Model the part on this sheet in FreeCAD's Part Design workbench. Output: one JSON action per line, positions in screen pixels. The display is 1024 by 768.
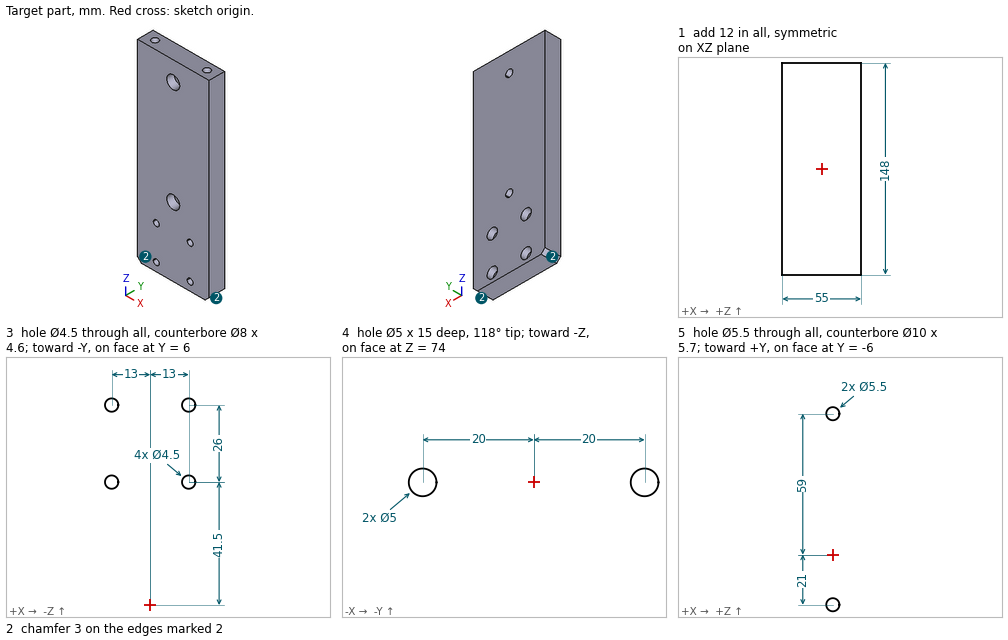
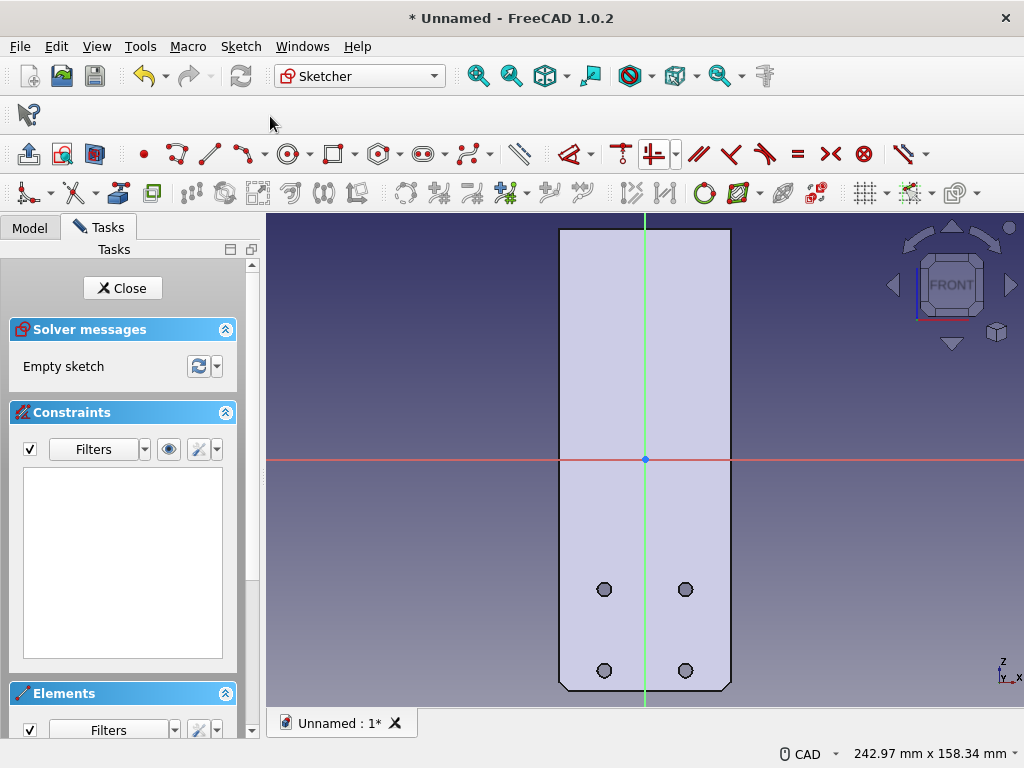
{"action": "key", "text": "g c"}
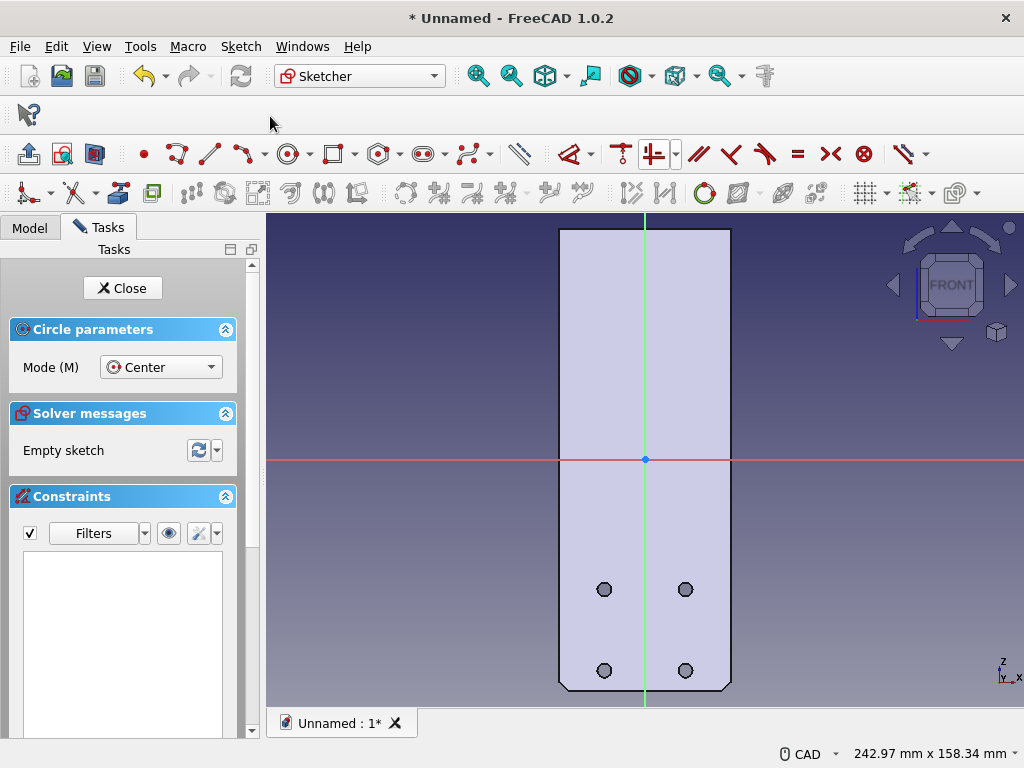
{"action": "scroll", "coordinate": [645, 276], "scroll_direction": "up", "scroll_amount": 5}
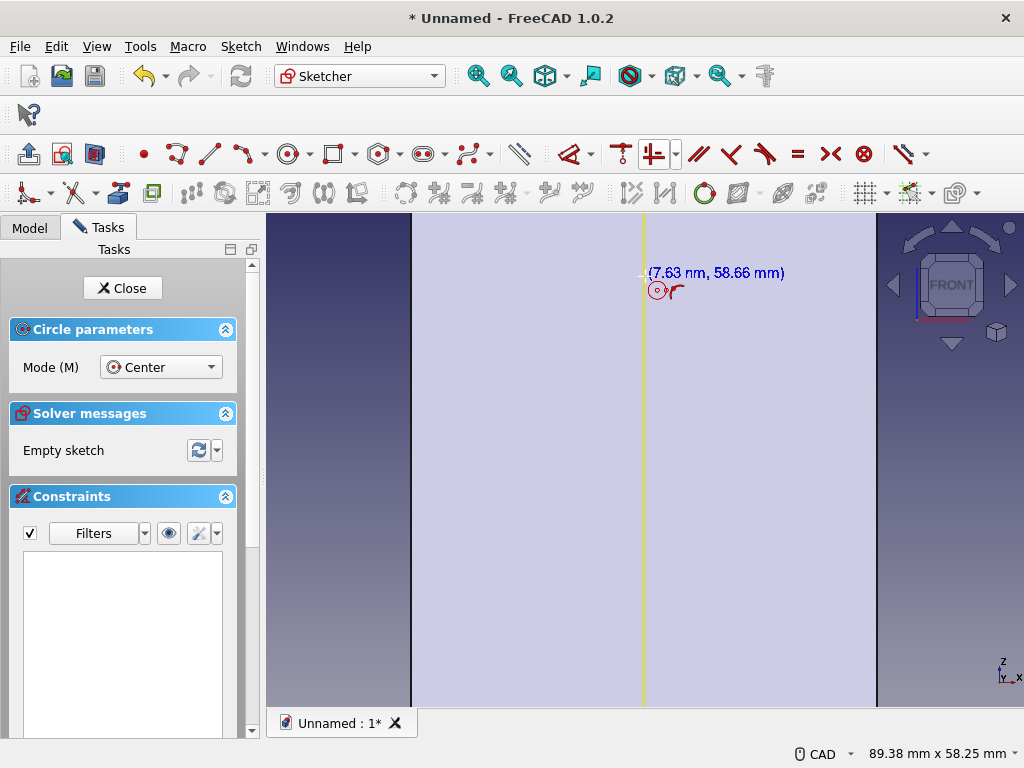
{"action": "left_click", "coordinate": [644, 276]}
{"action": "mouse_move", "coordinate": [661, 259]}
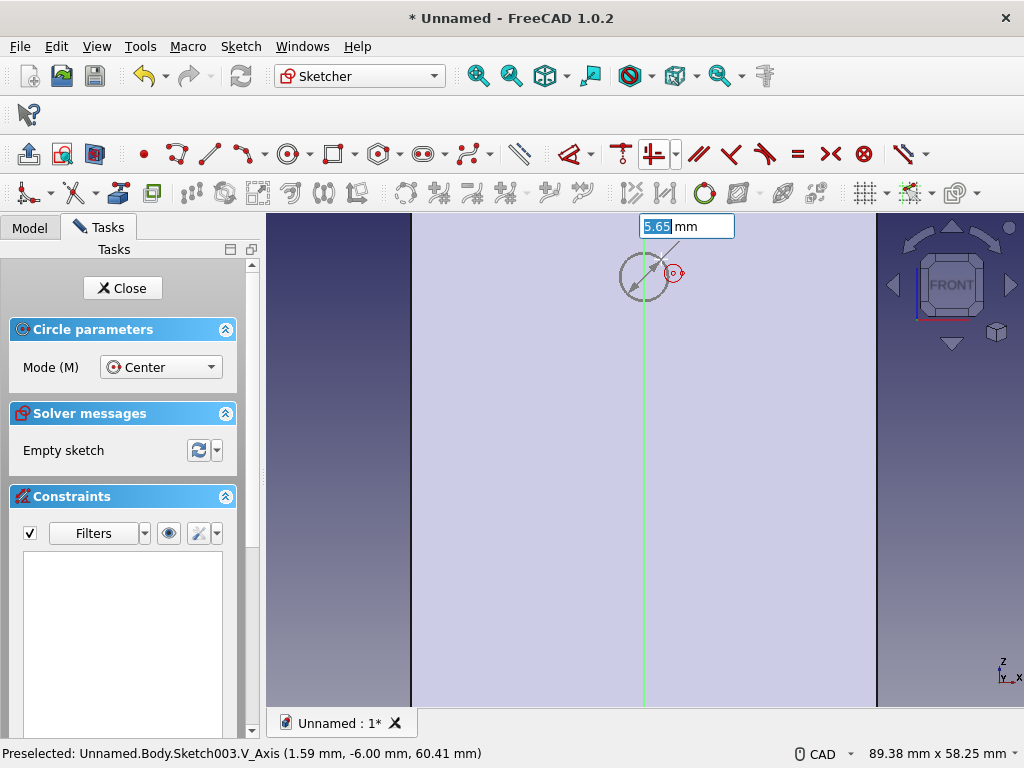
{"action": "type", "text": "5.5"}
{"action": "key", "text": "Return"}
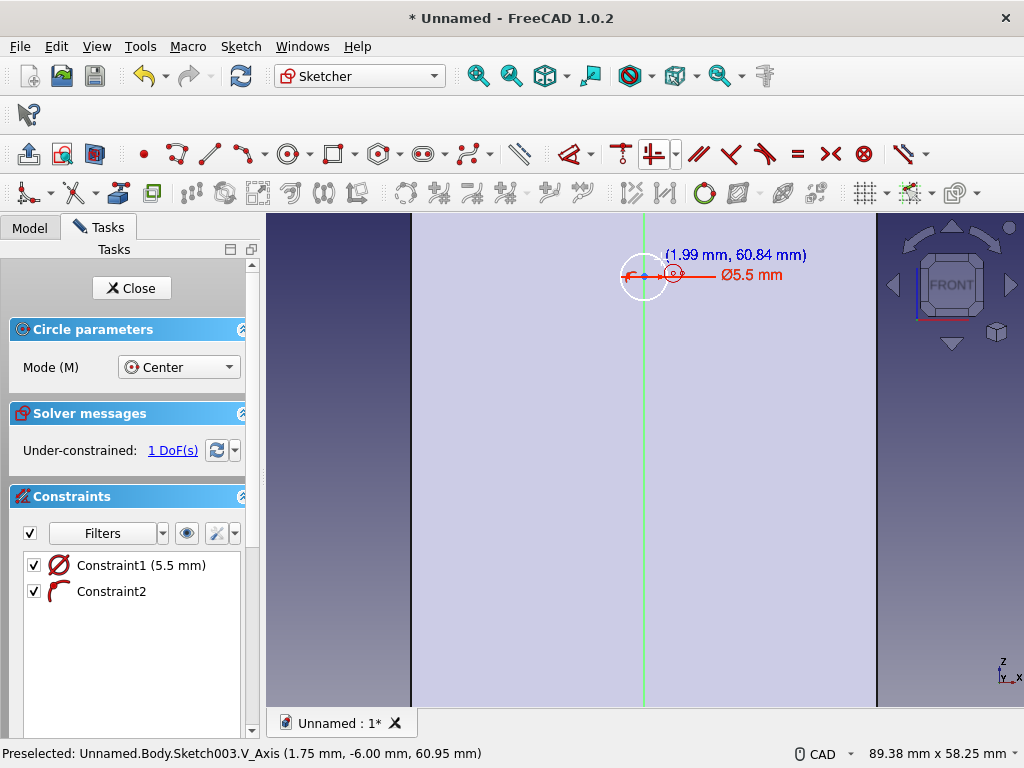
{"action": "scroll", "coordinate": [521, 334], "scroll_direction": "down", "scroll_amount": 4}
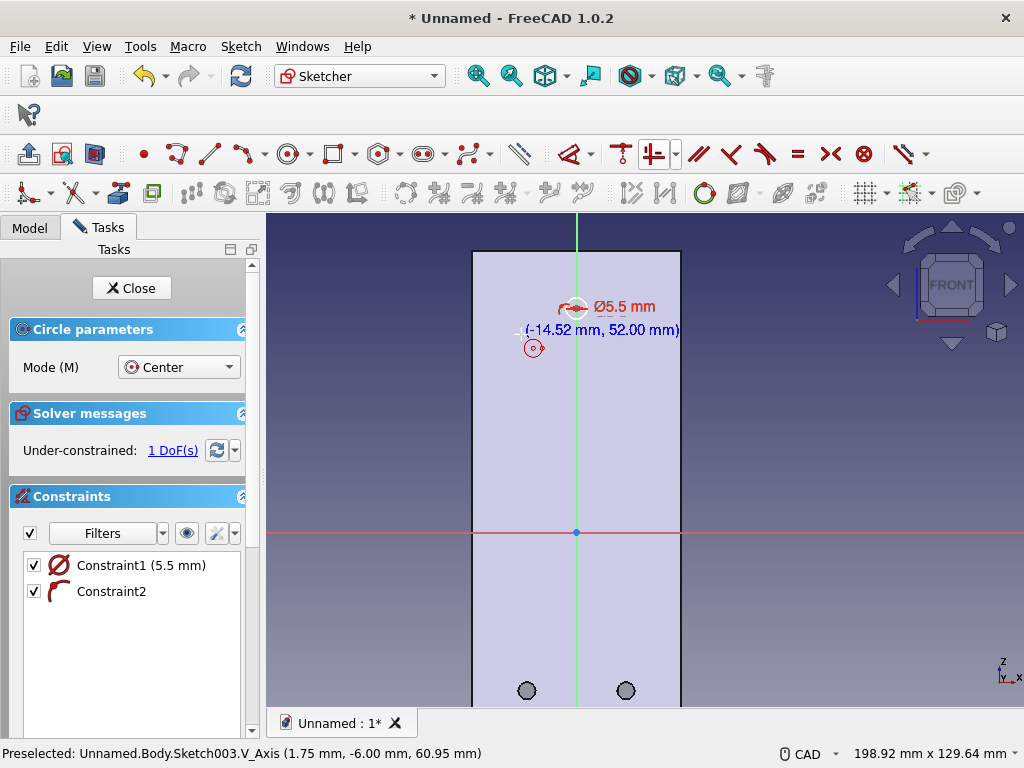
{"action": "scroll", "coordinate": [577, 613], "scroll_direction": "up", "scroll_amount": 4}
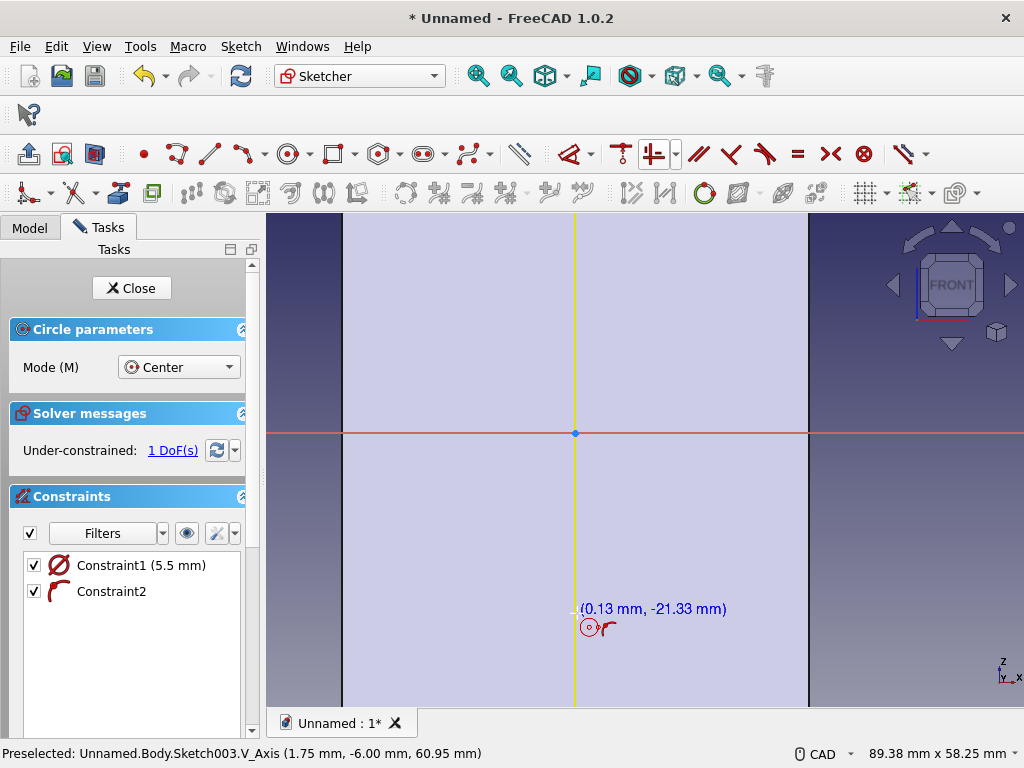
{"action": "left_click", "coordinate": [575, 611]}
{"action": "mouse_move", "coordinate": [592, 595]}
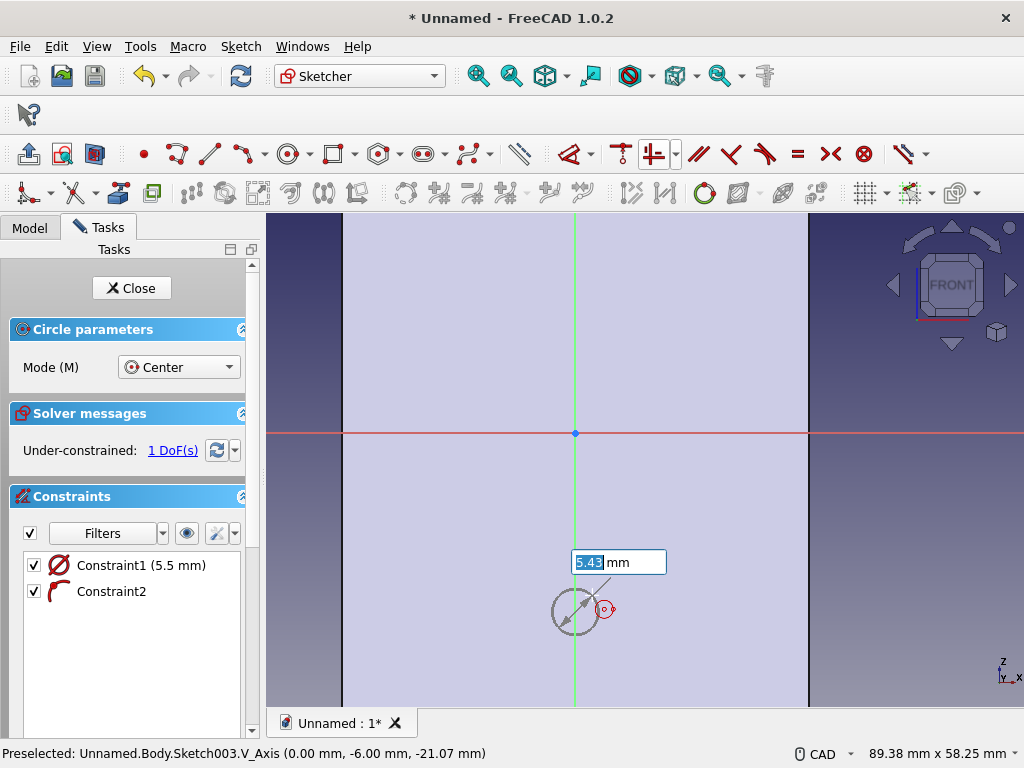
{"action": "type", "text": "5.5"}
{"action": "key", "text": "Return"}
{"action": "key", "text": "Escape"}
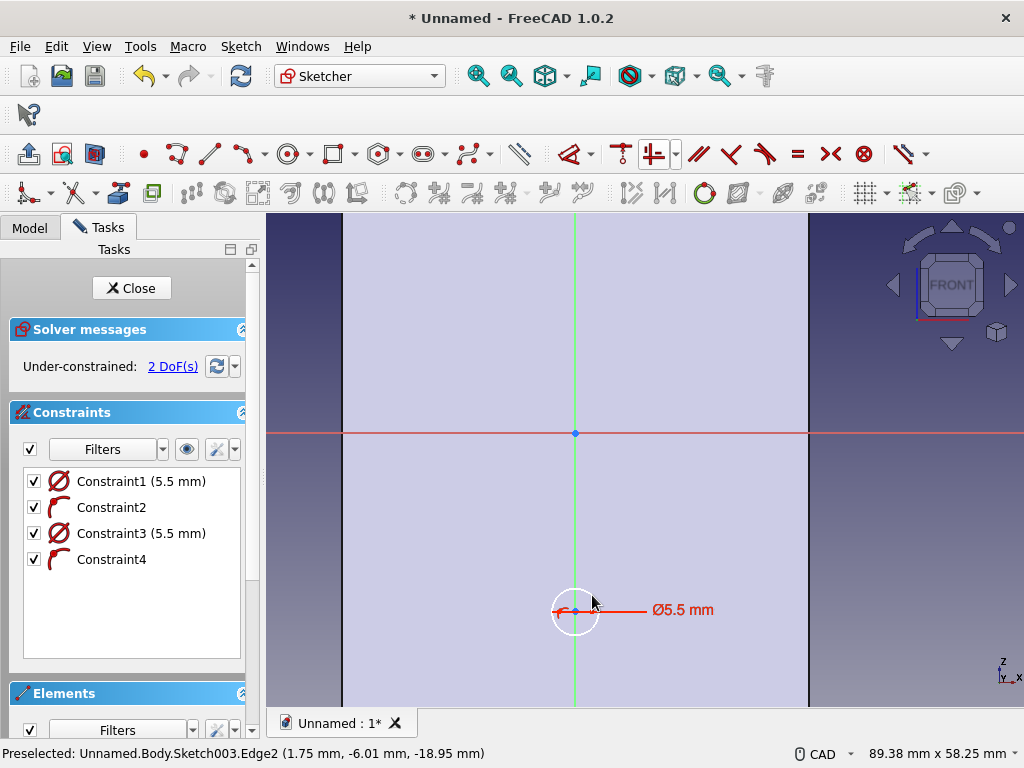
{"action": "key", "text": "d"}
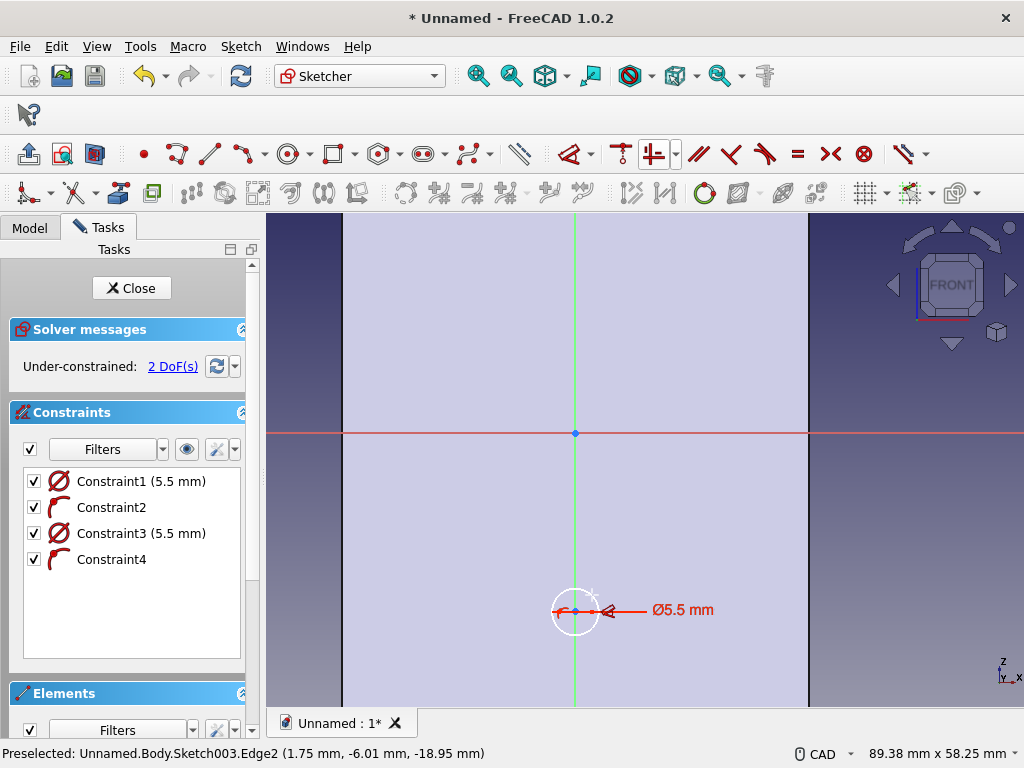
{"action": "scroll", "coordinate": [577, 613], "scroll_direction": "down", "scroll_amount": 4}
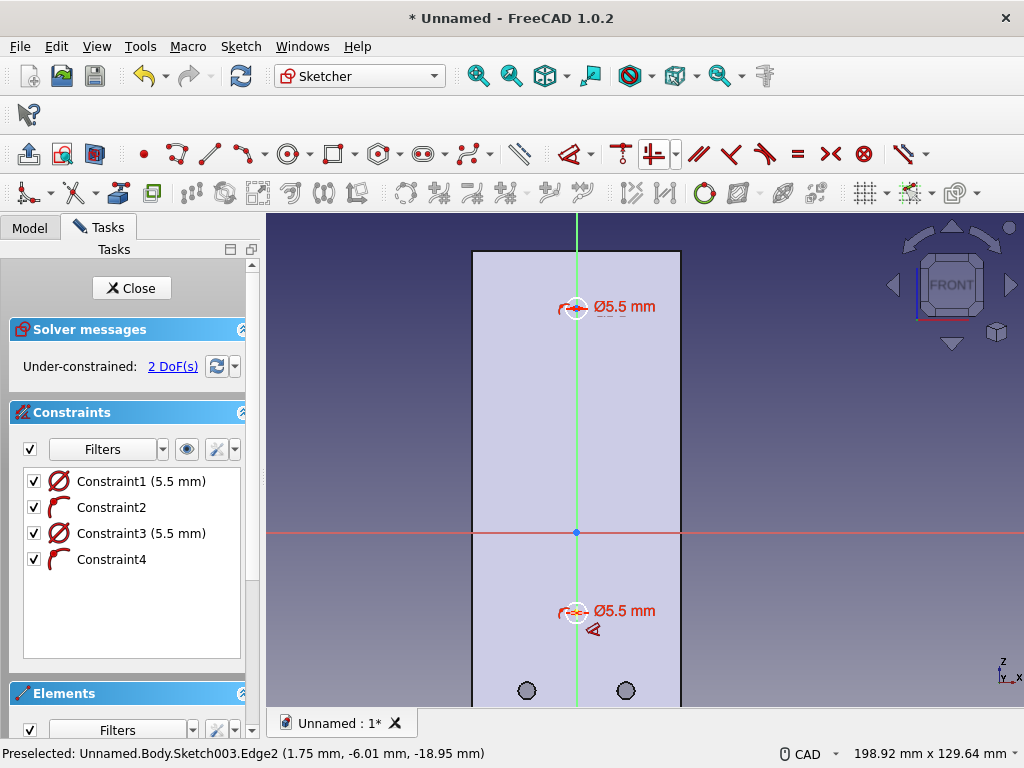
{"action": "left_click", "coordinate": [577, 309]}
{"action": "left_click", "coordinate": [611, 421]}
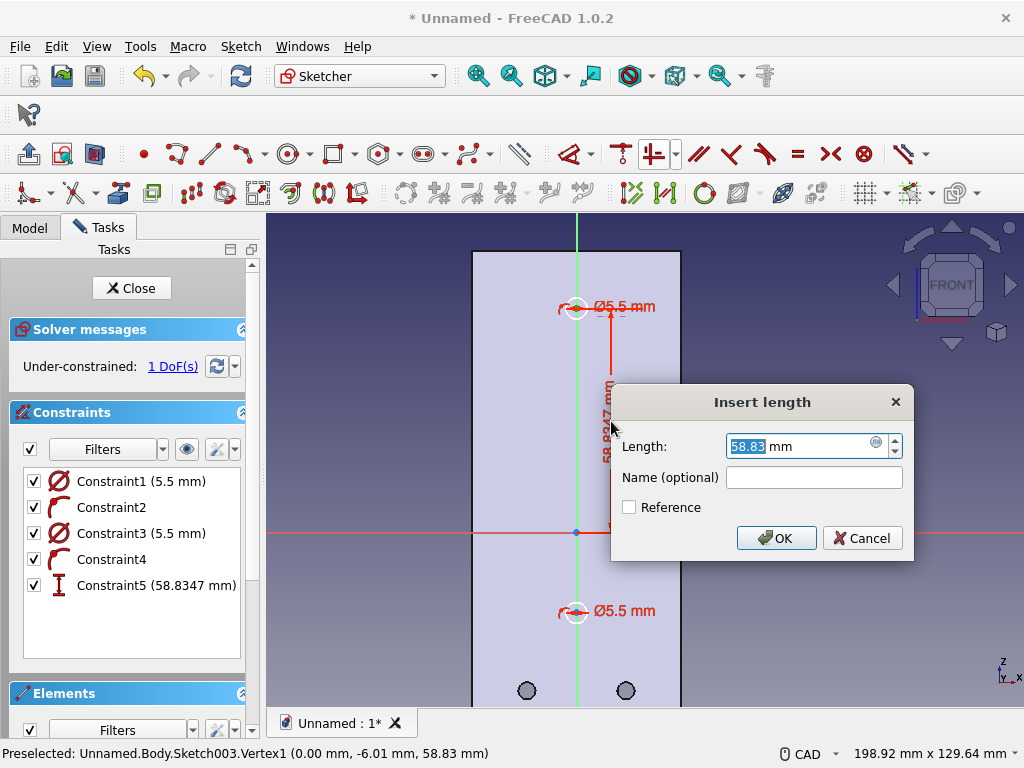
{"action": "type", "text": "59"}
{"action": "key", "text": "Return"}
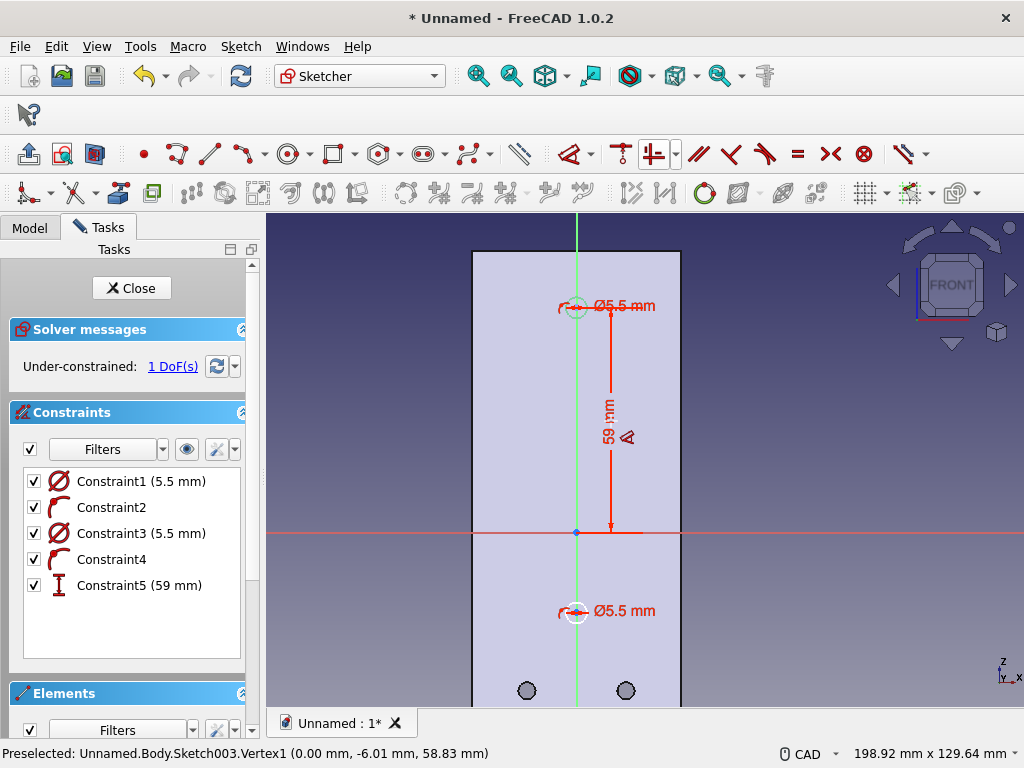
{"action": "left_click", "coordinate": [577, 613]}
{"action": "left_click", "coordinate": [611, 573]}